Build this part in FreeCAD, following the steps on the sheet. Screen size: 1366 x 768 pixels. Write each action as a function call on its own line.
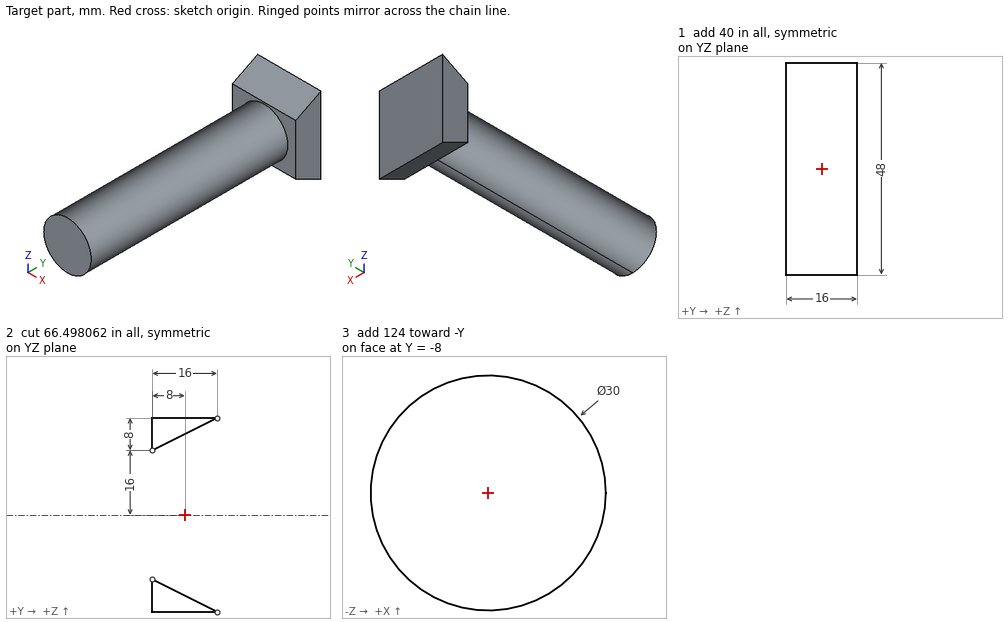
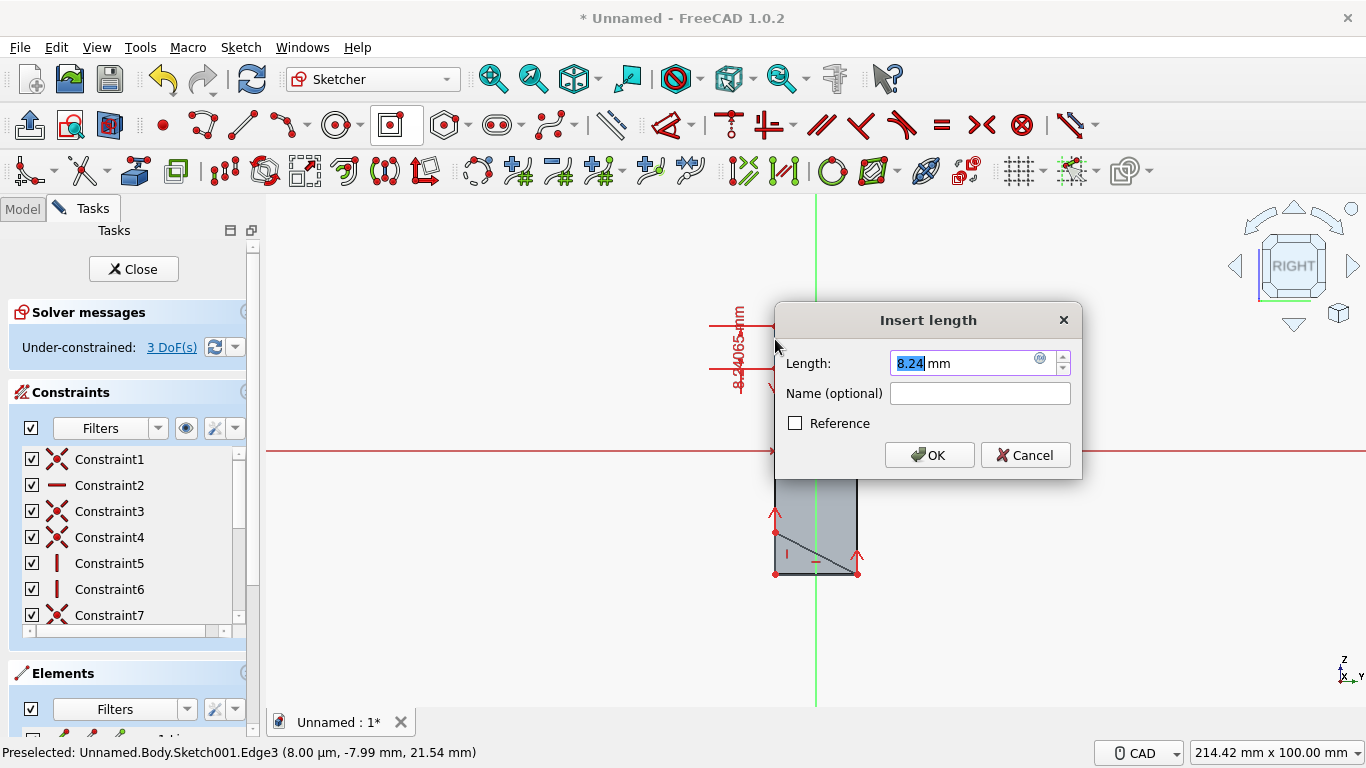
text(8)
key(Return)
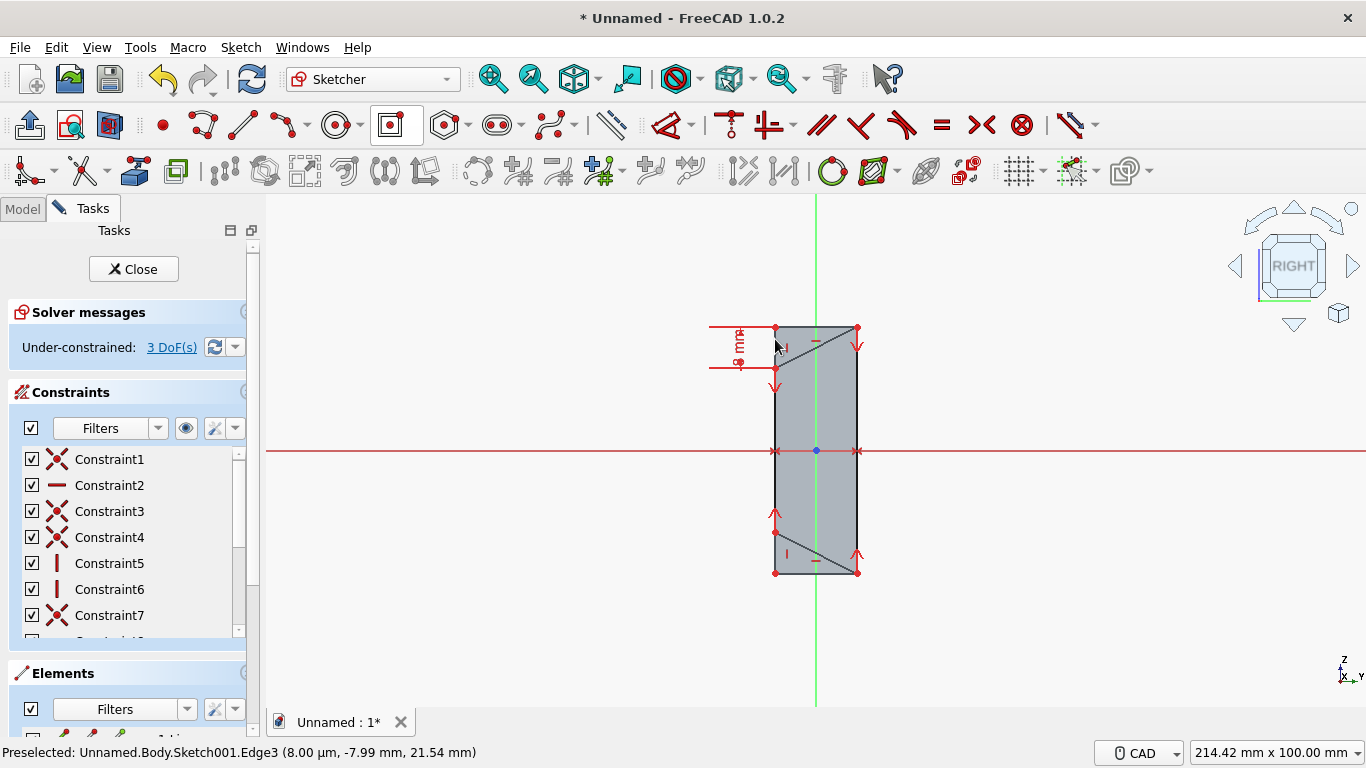
scroll(832, 327, up, 2)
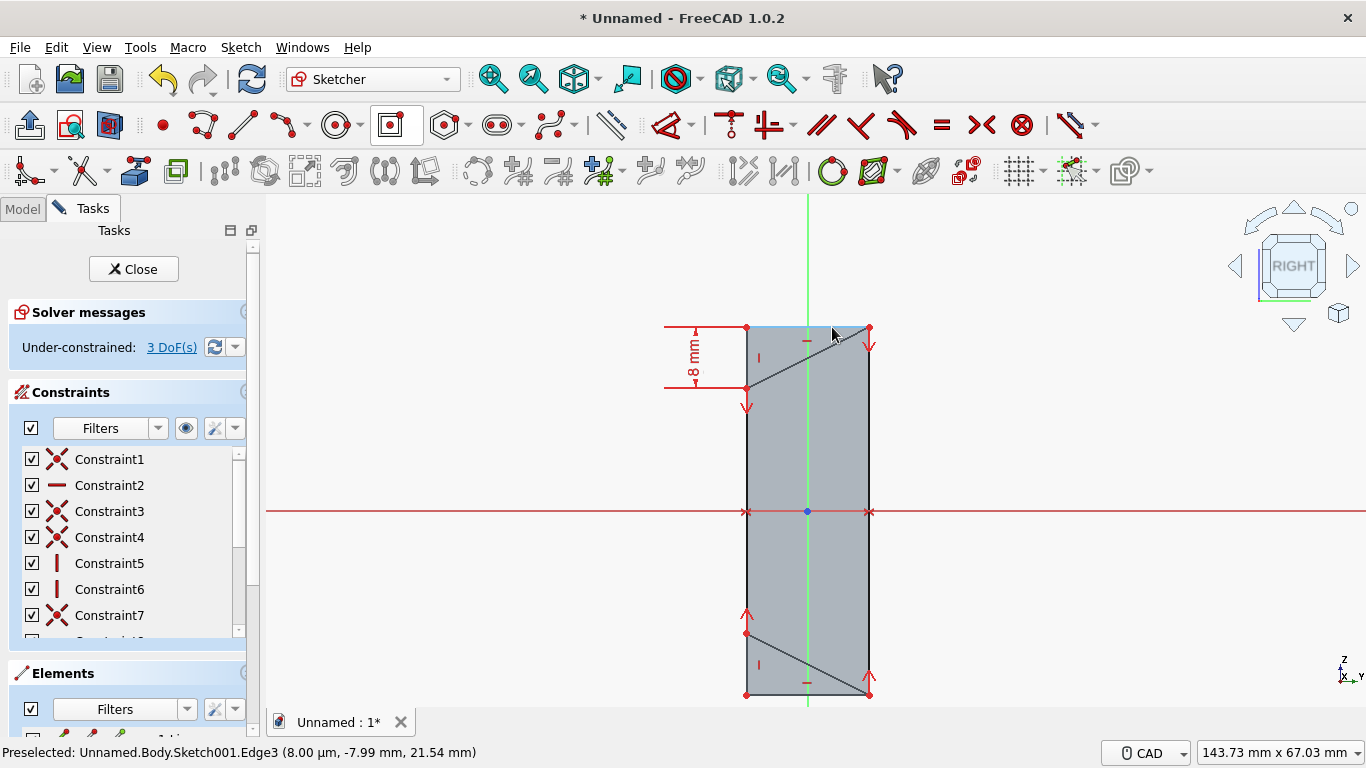
click(832, 327)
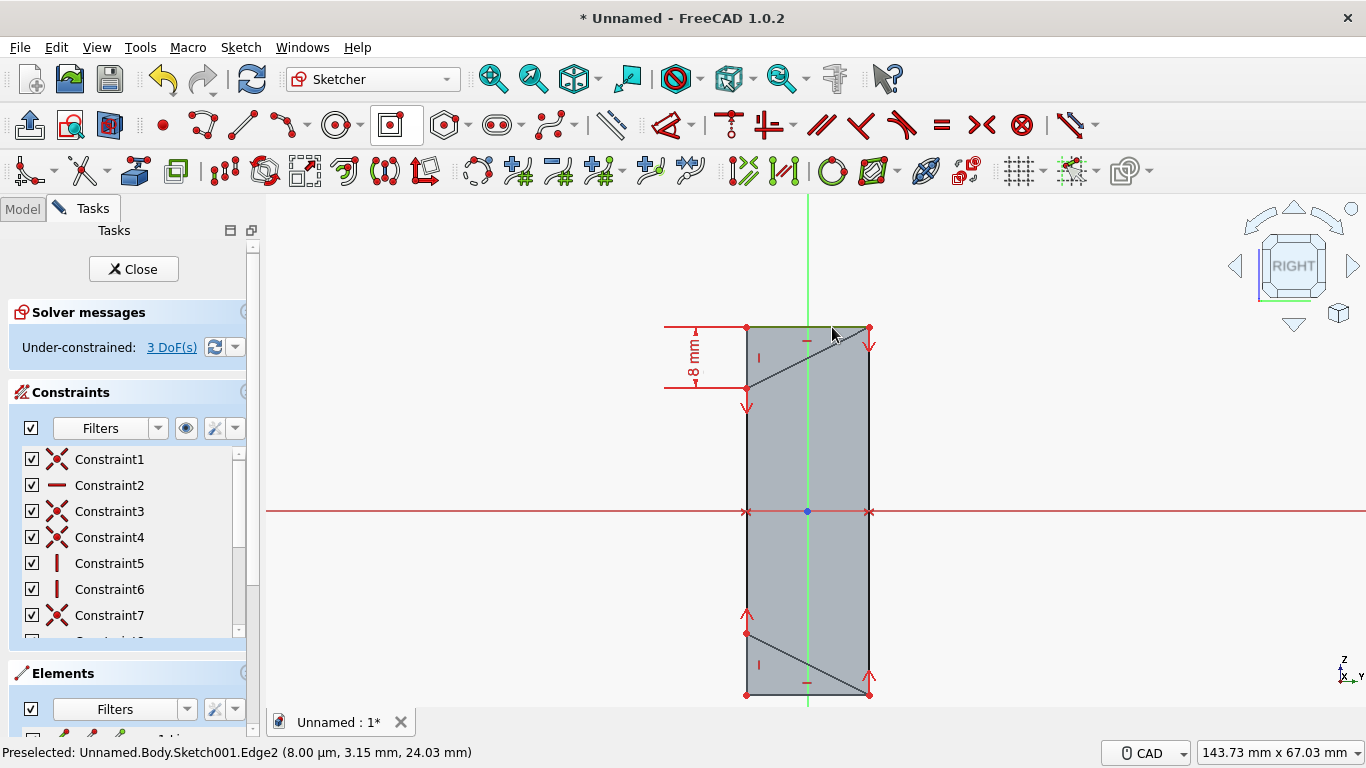
key(l)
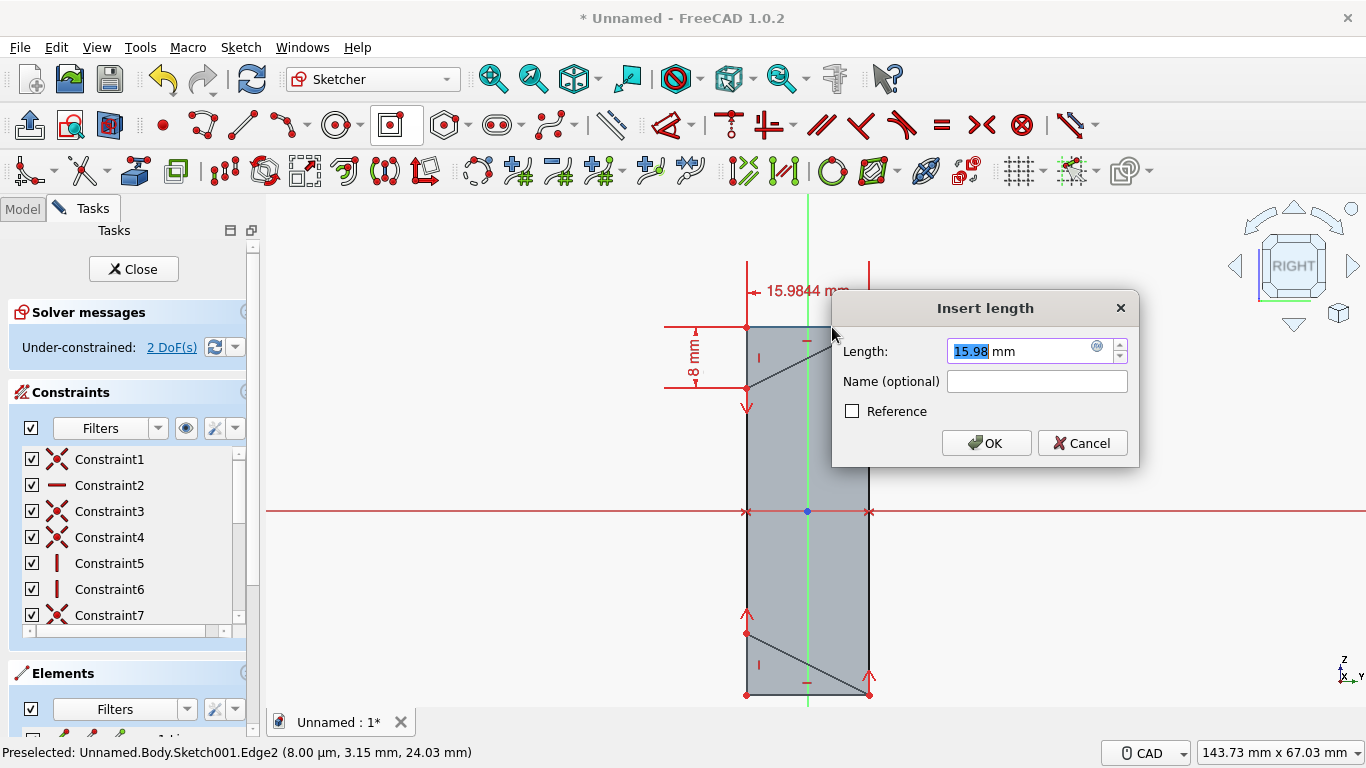
text(16)
key(Return)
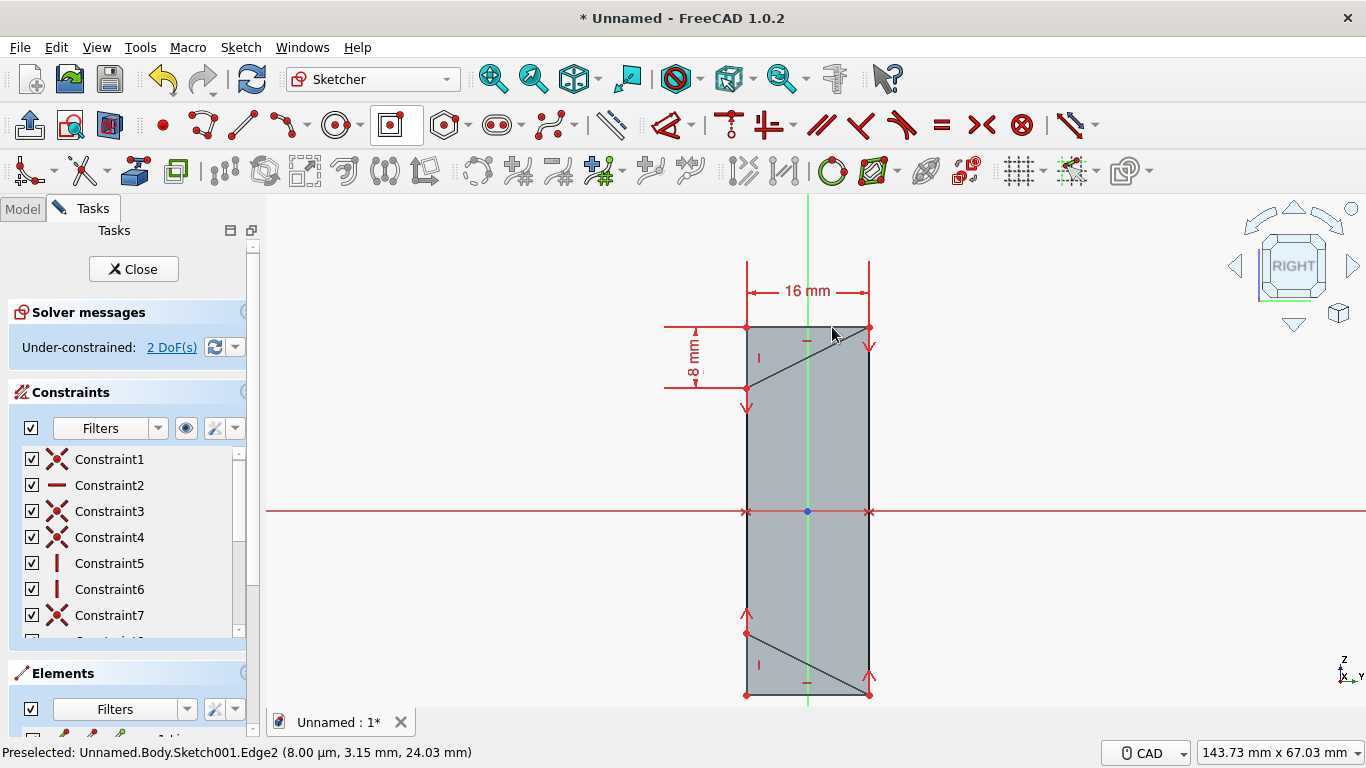
click(747, 388)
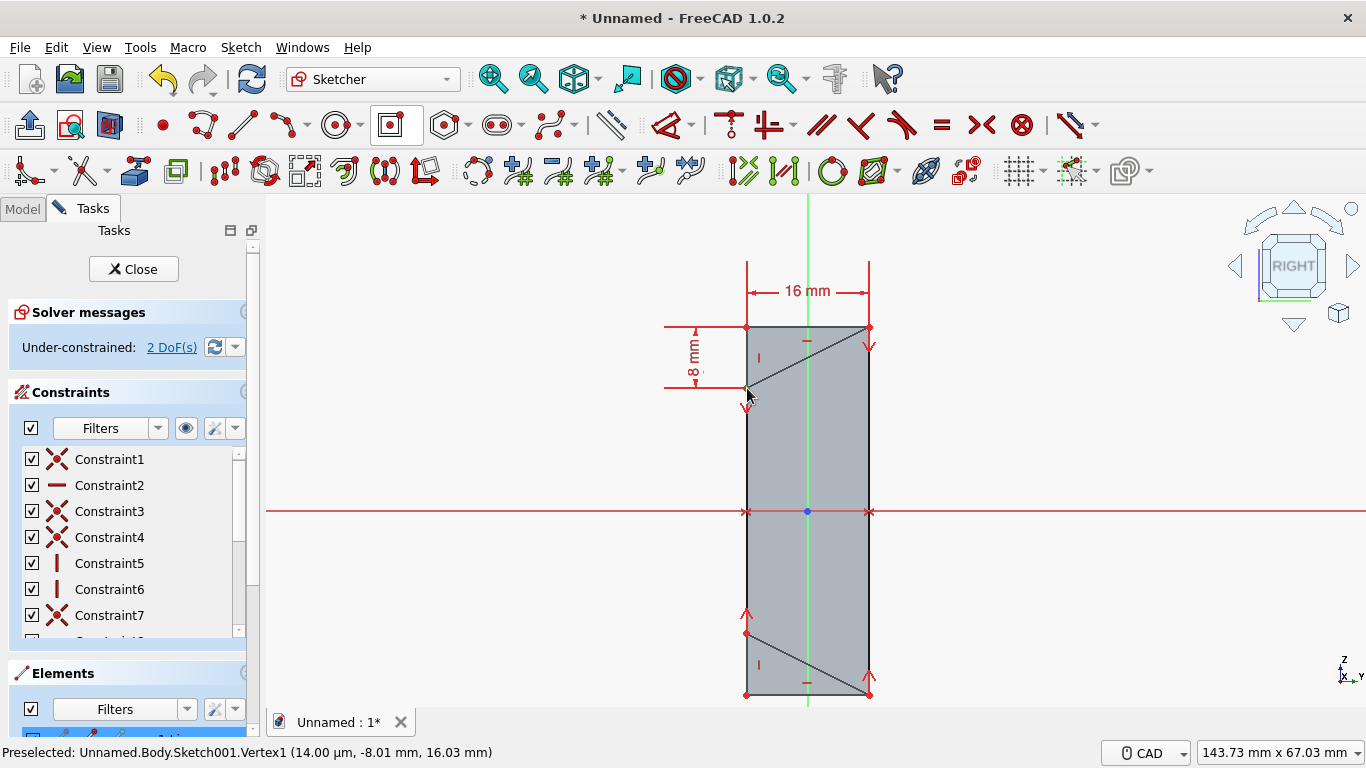
key(l)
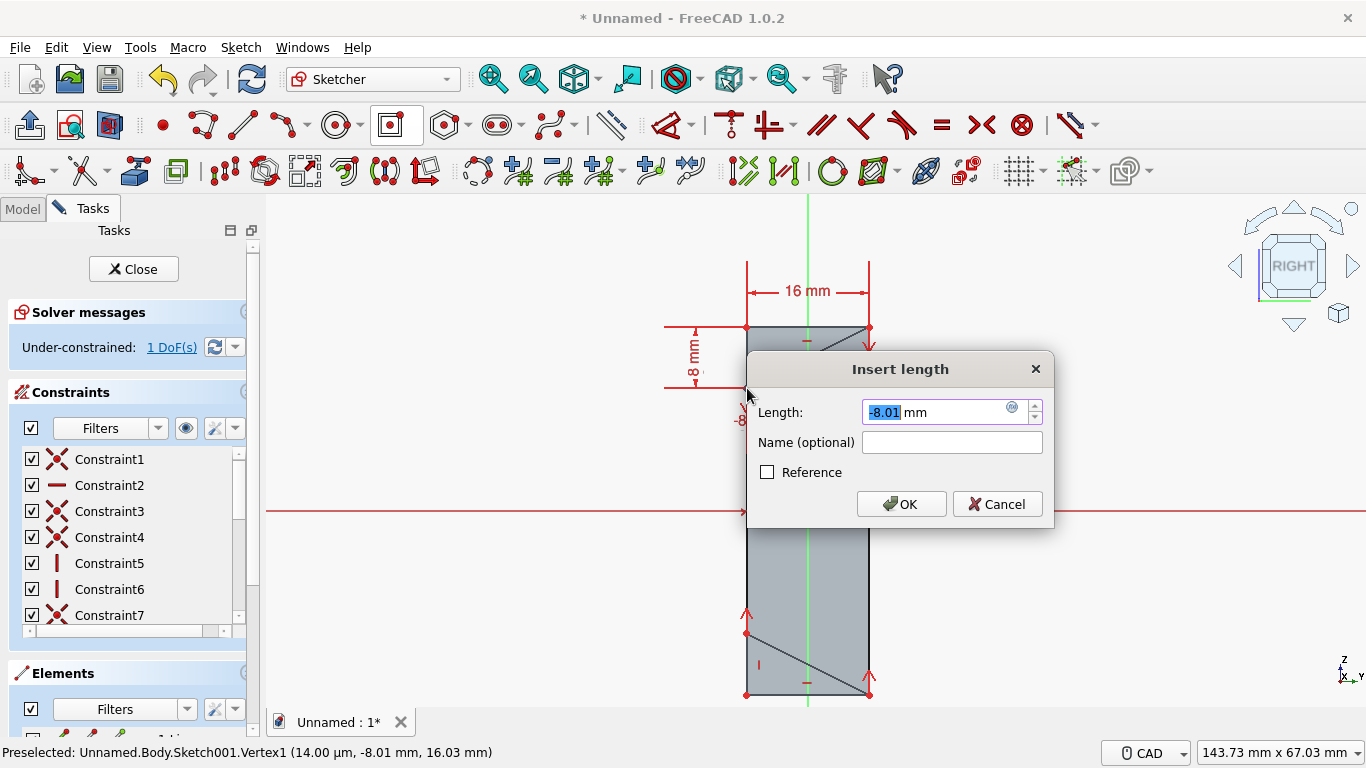
text(-8)
key(Return)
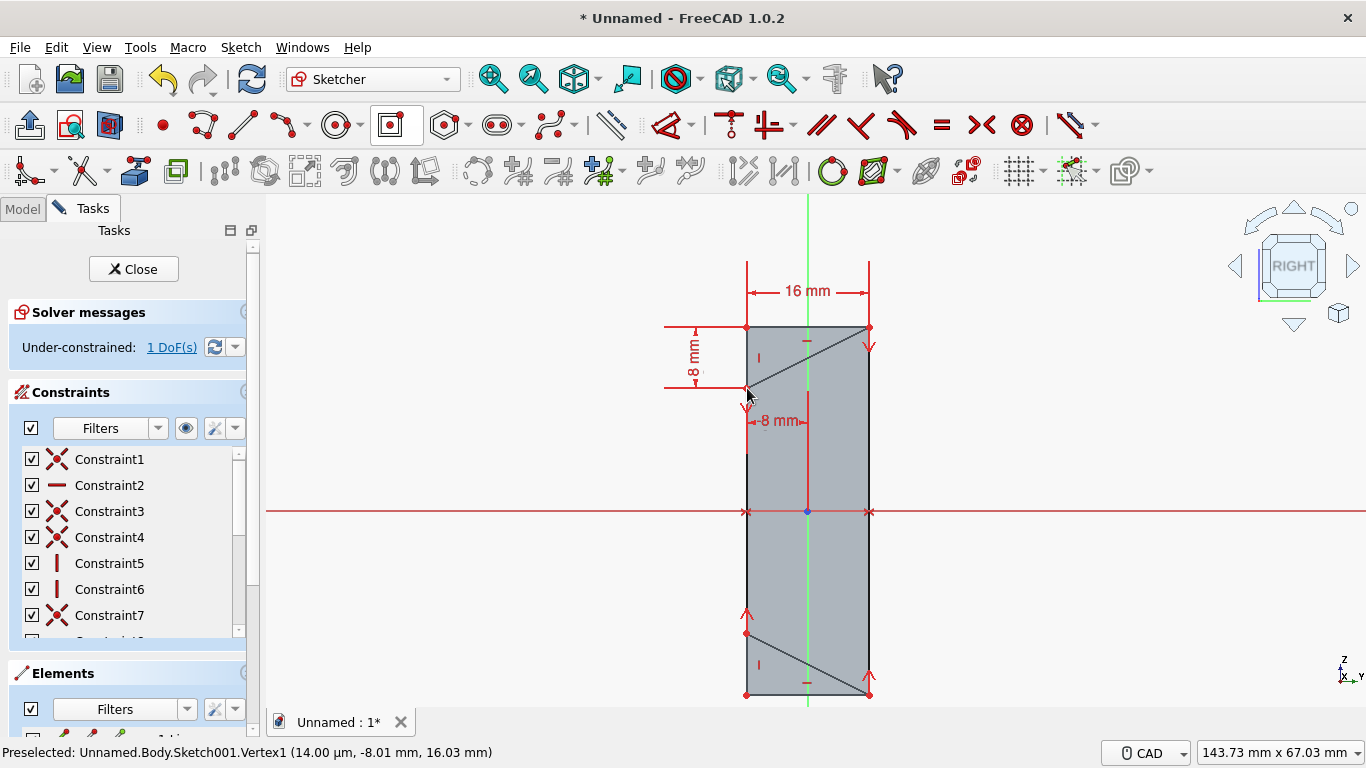
click(747, 388)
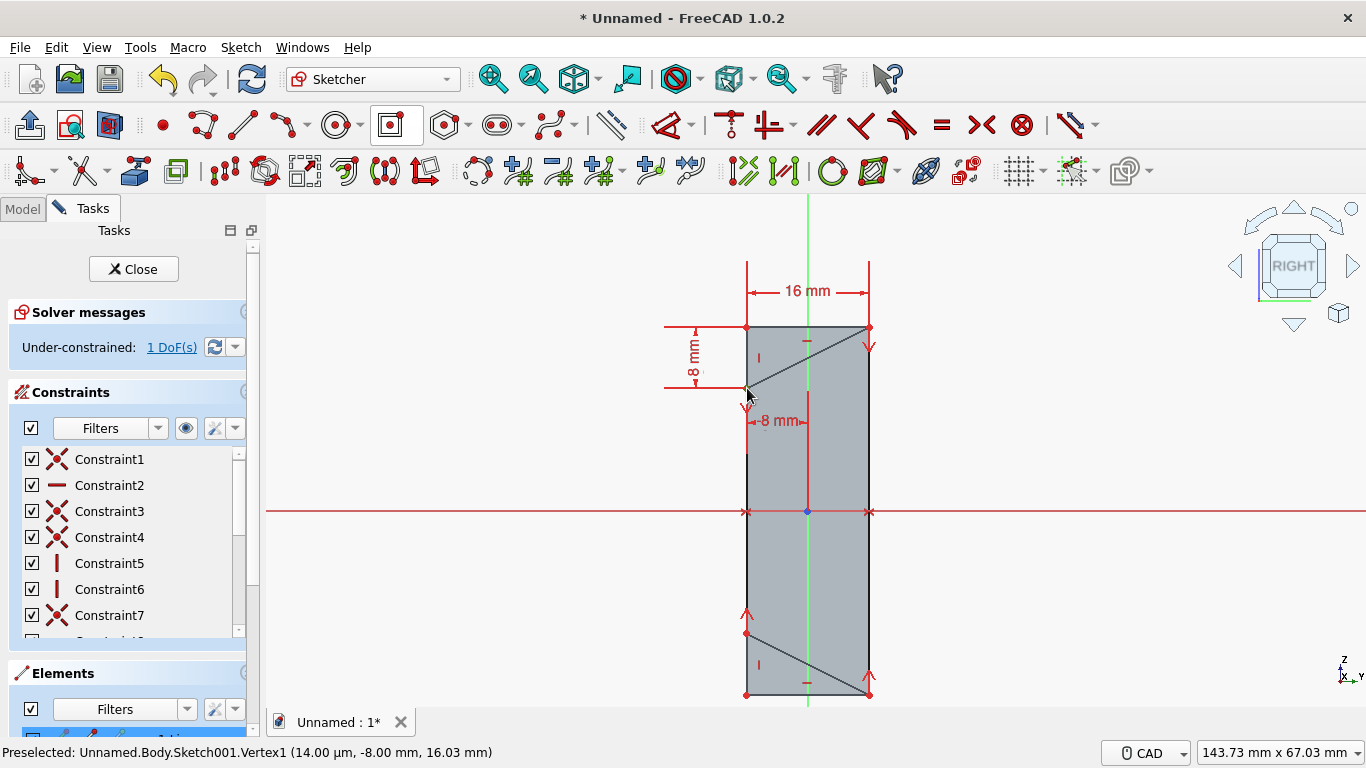
click(694, 126)